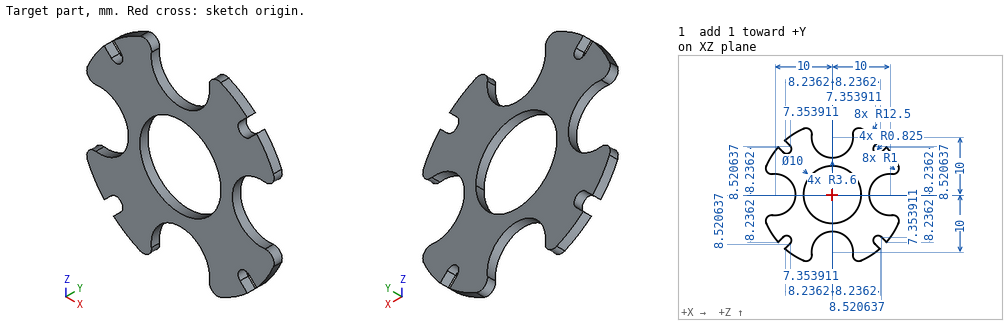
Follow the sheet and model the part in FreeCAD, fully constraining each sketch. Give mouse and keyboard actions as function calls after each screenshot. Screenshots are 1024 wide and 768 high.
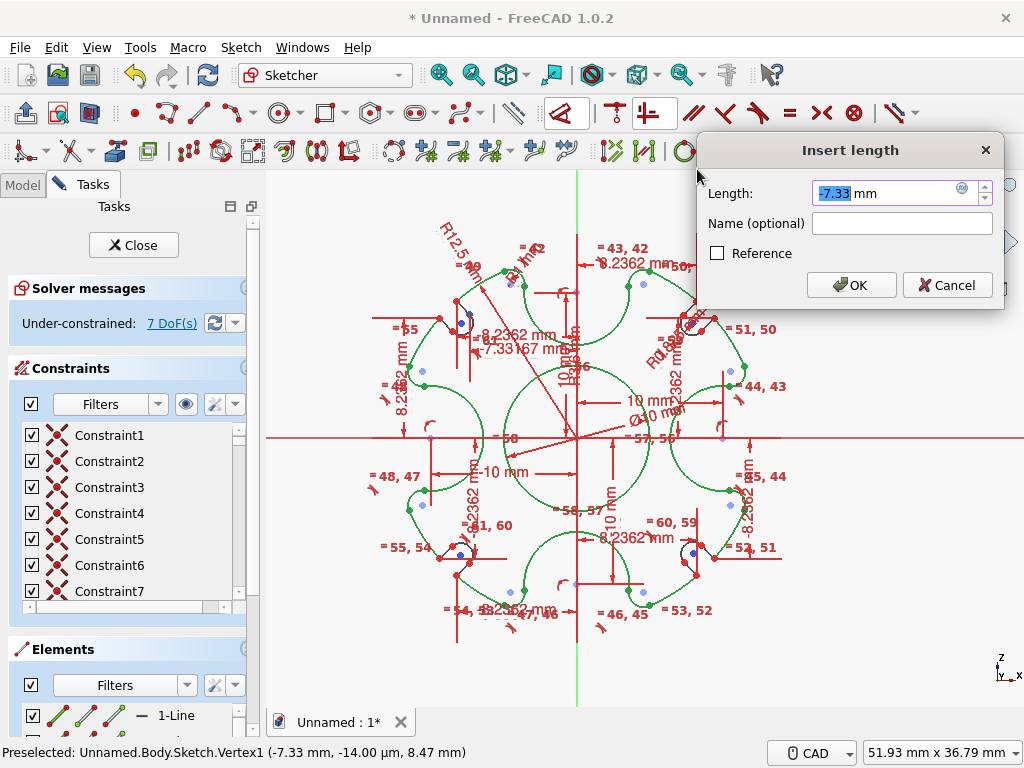
text(-7.353911)
key(Return)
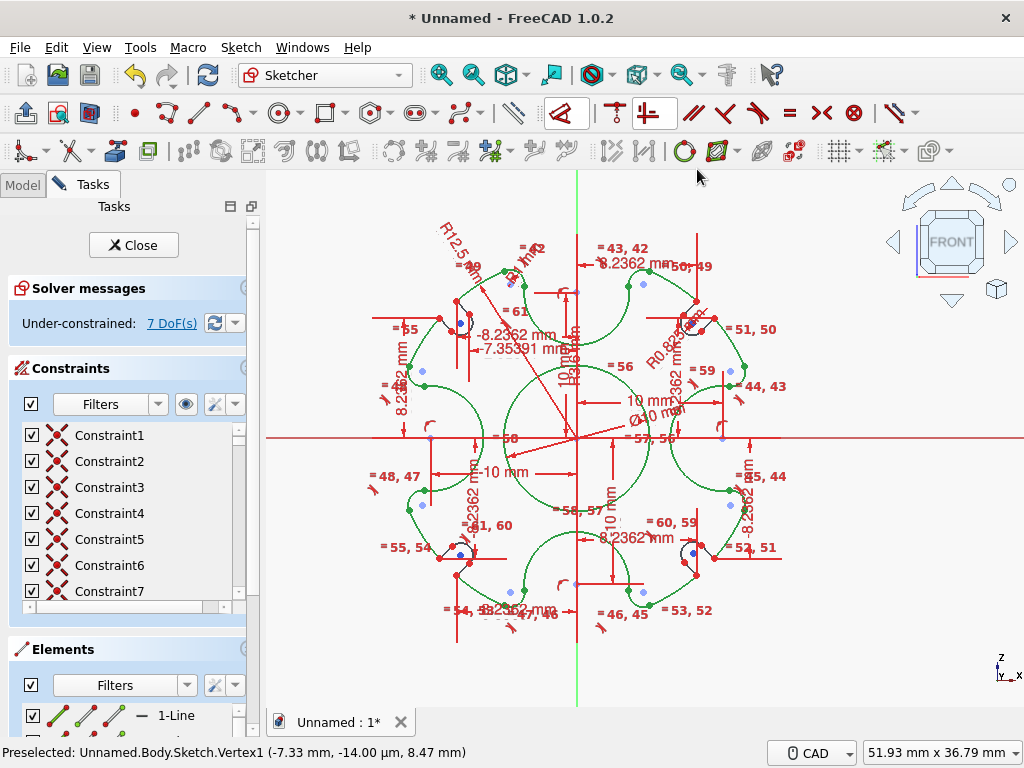
click(469, 315)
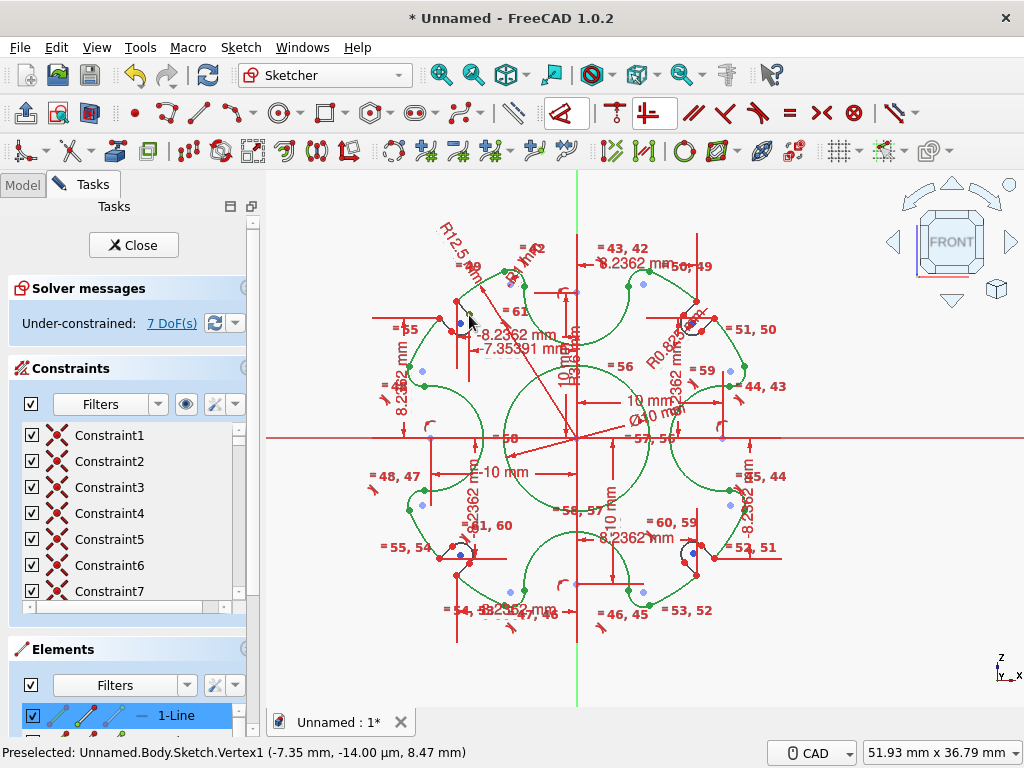
click(584, 114)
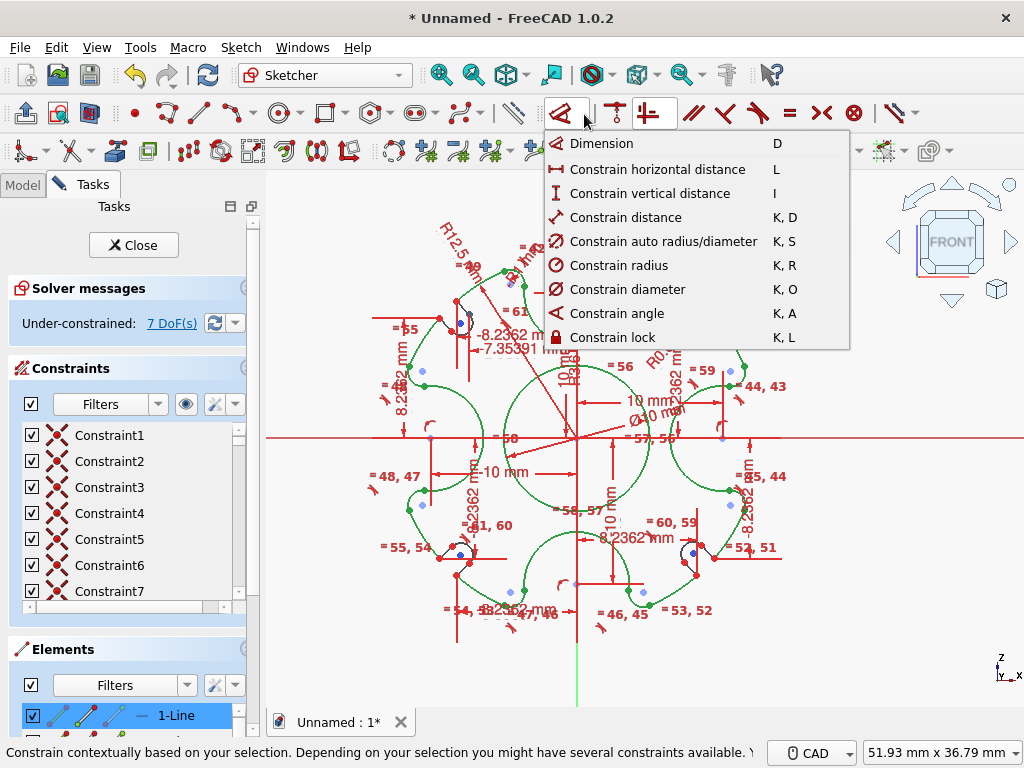
click(697, 193)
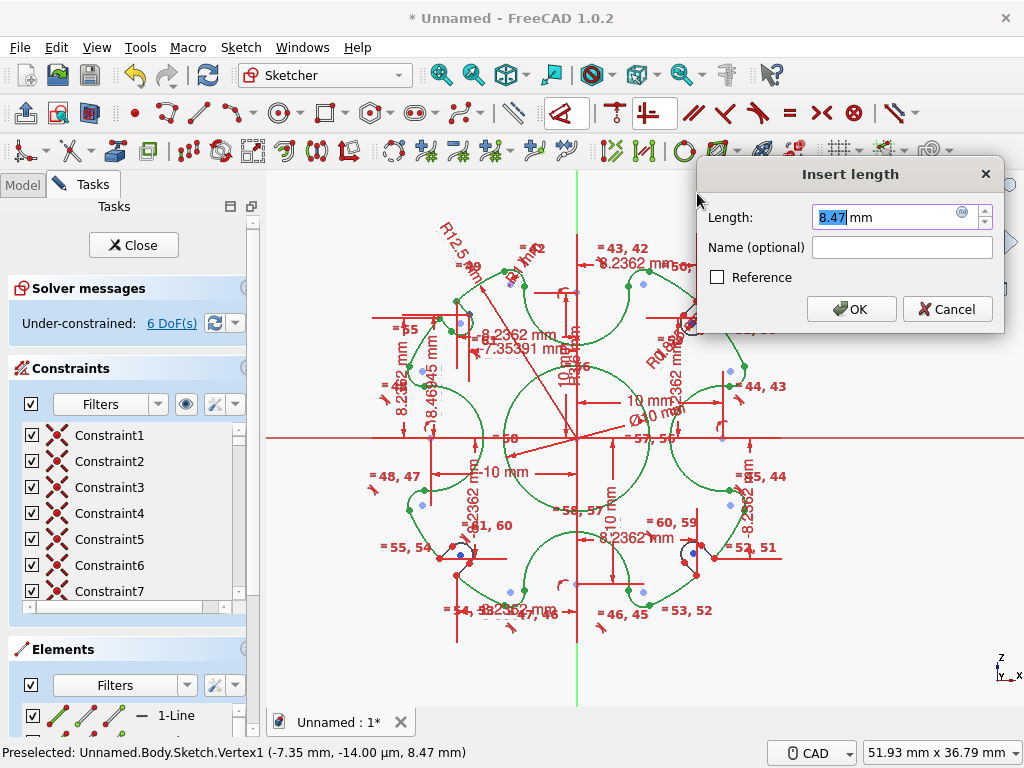
text(8.520637)
key(Return)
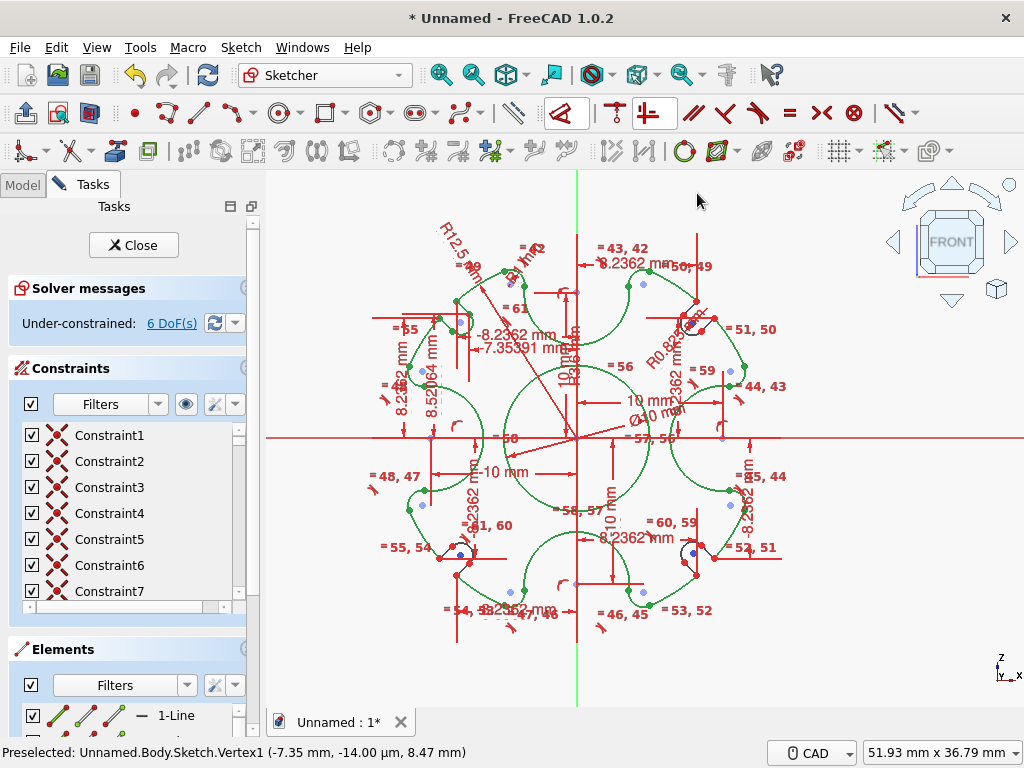
click(684, 315)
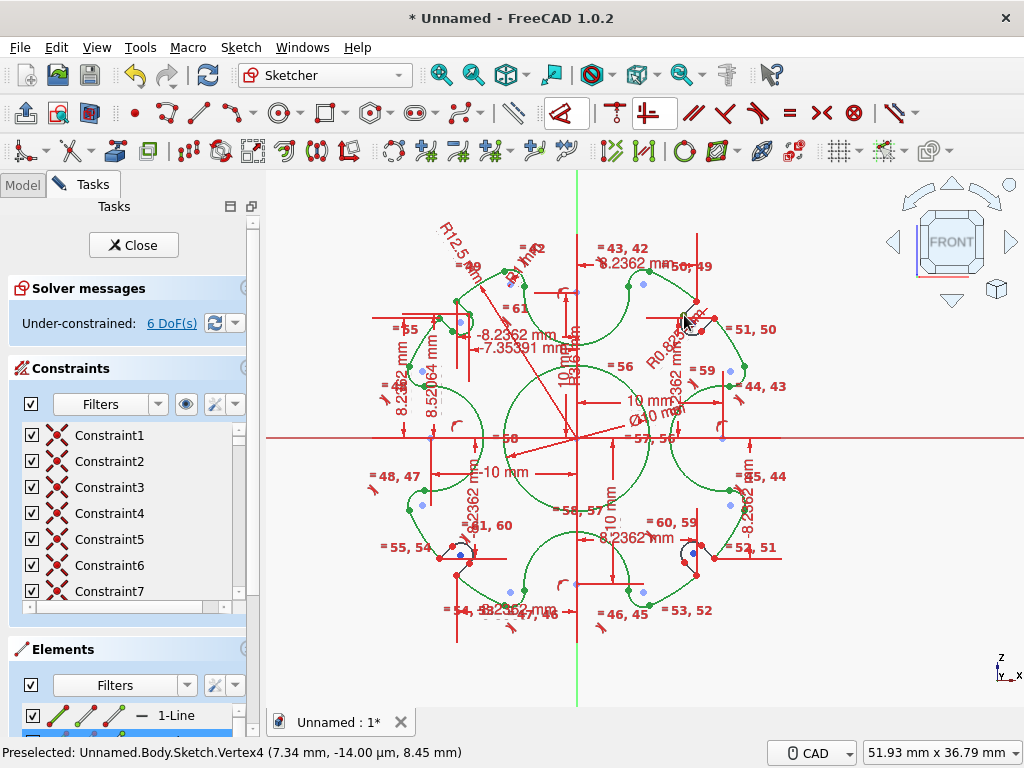
click(584, 114)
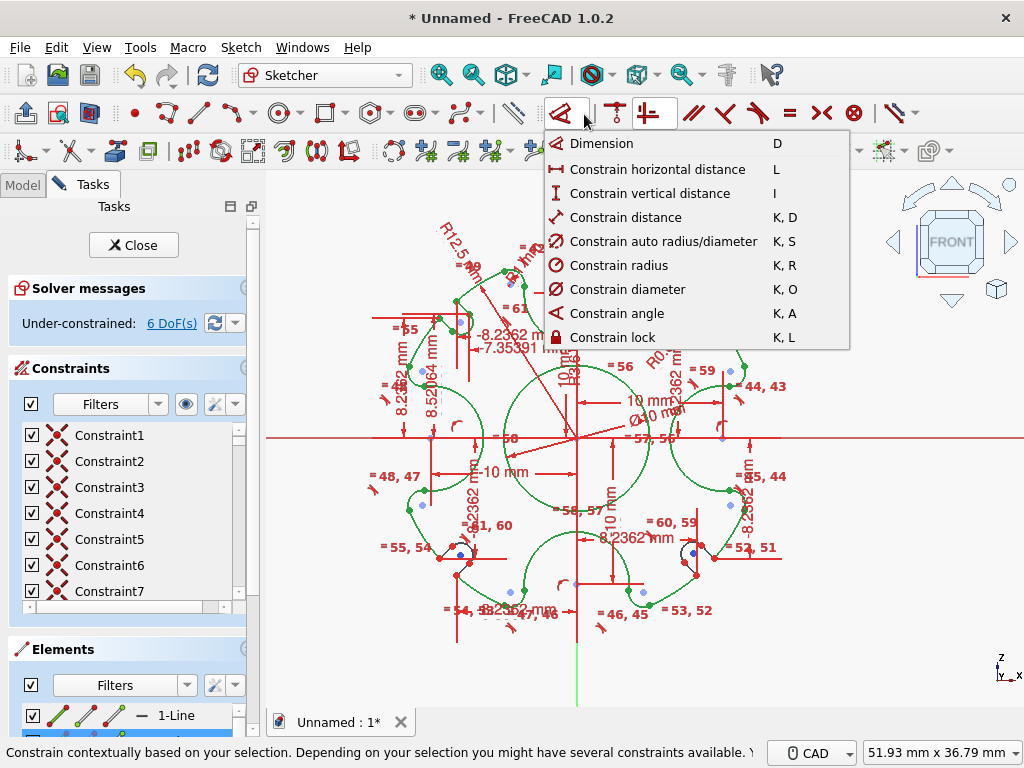
click(697, 169)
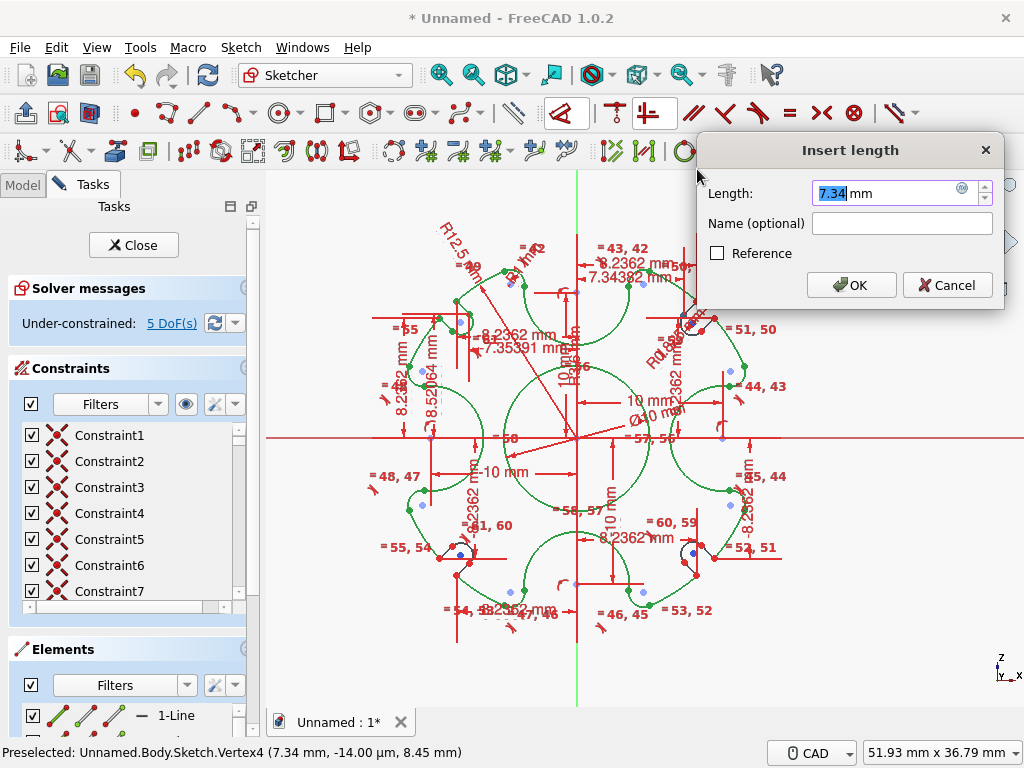
text(7.353911)
key(Return)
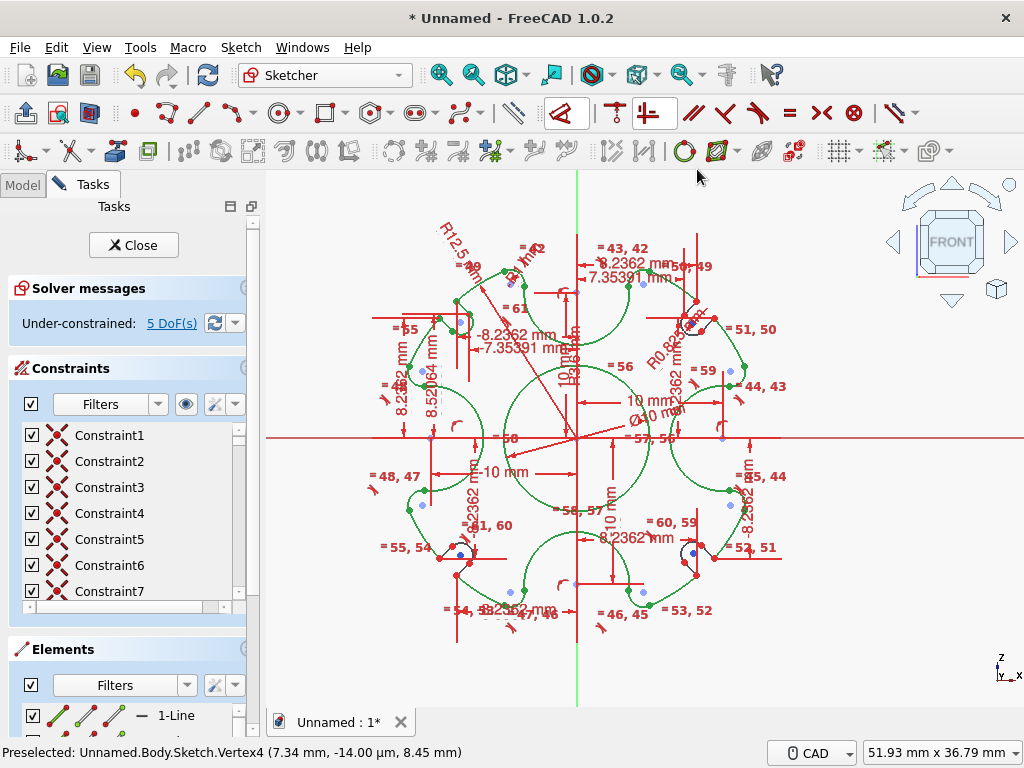
click(684, 315)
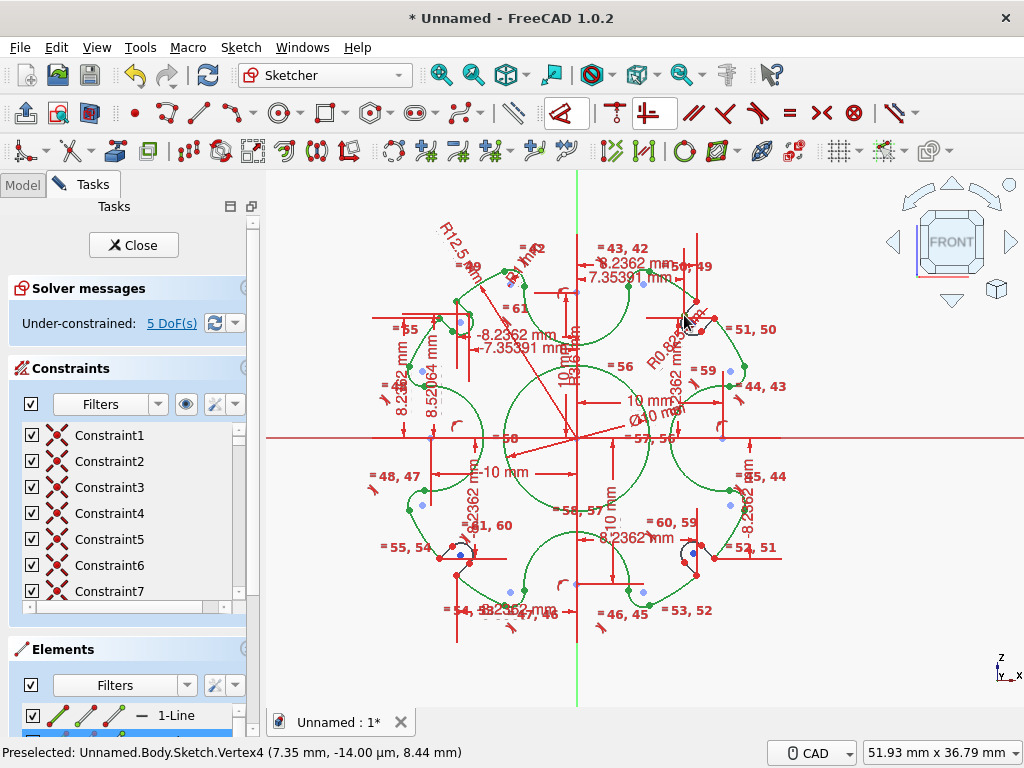
key(i)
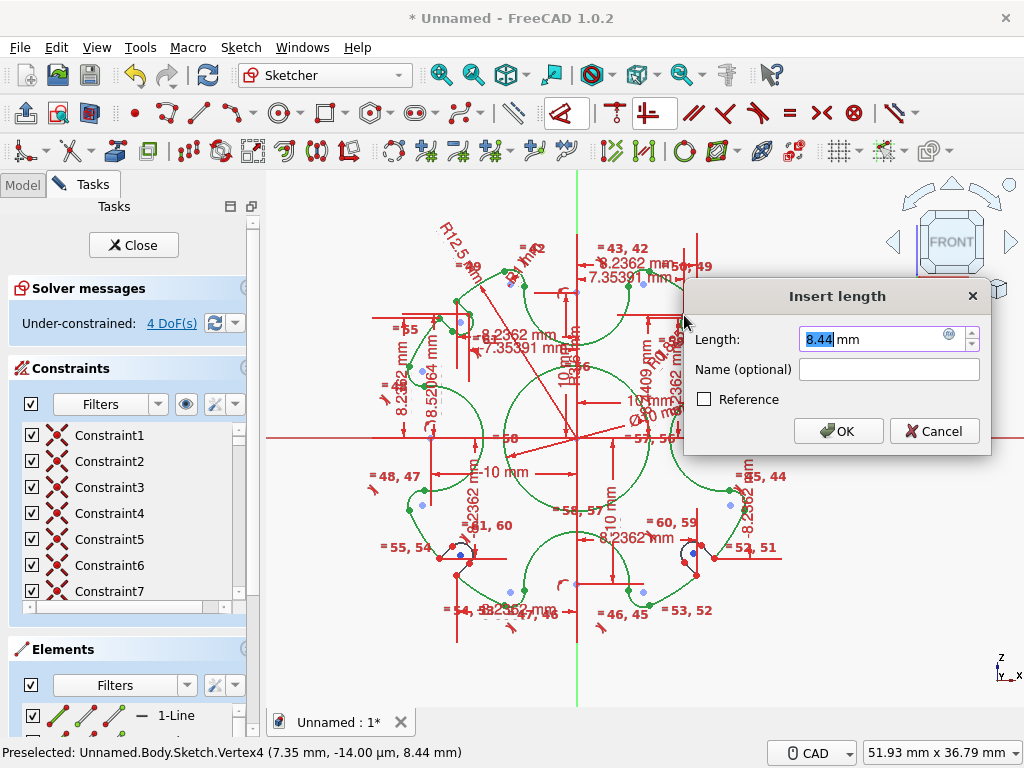
text(8.520637)
key(Return)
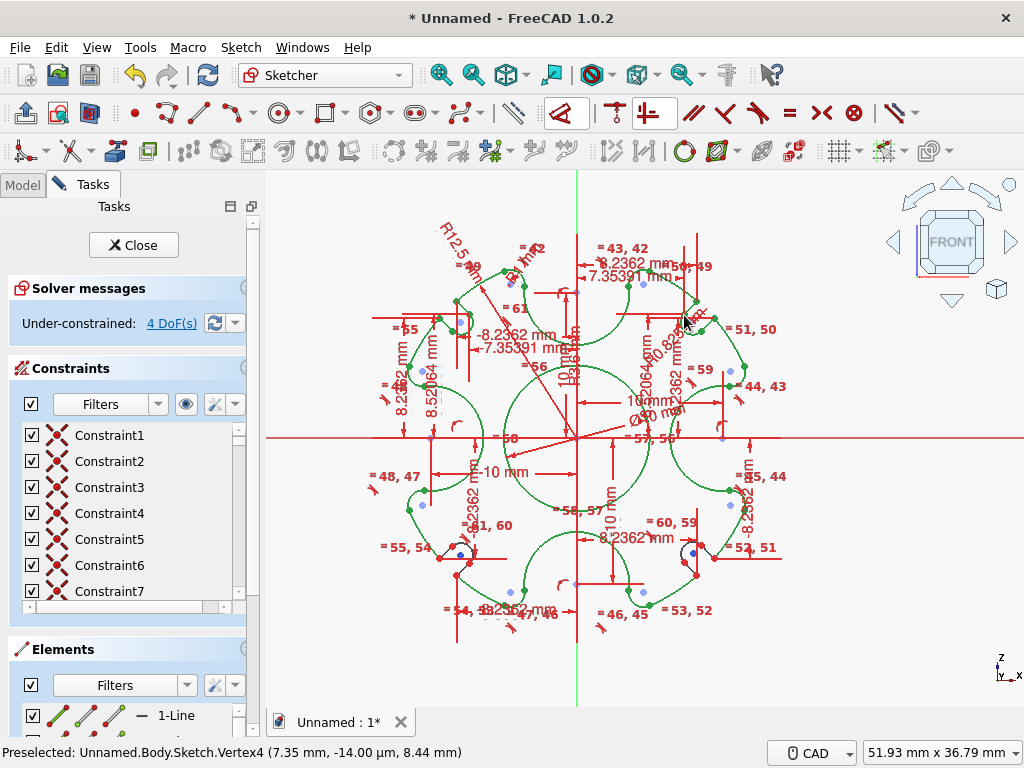
click(702, 546)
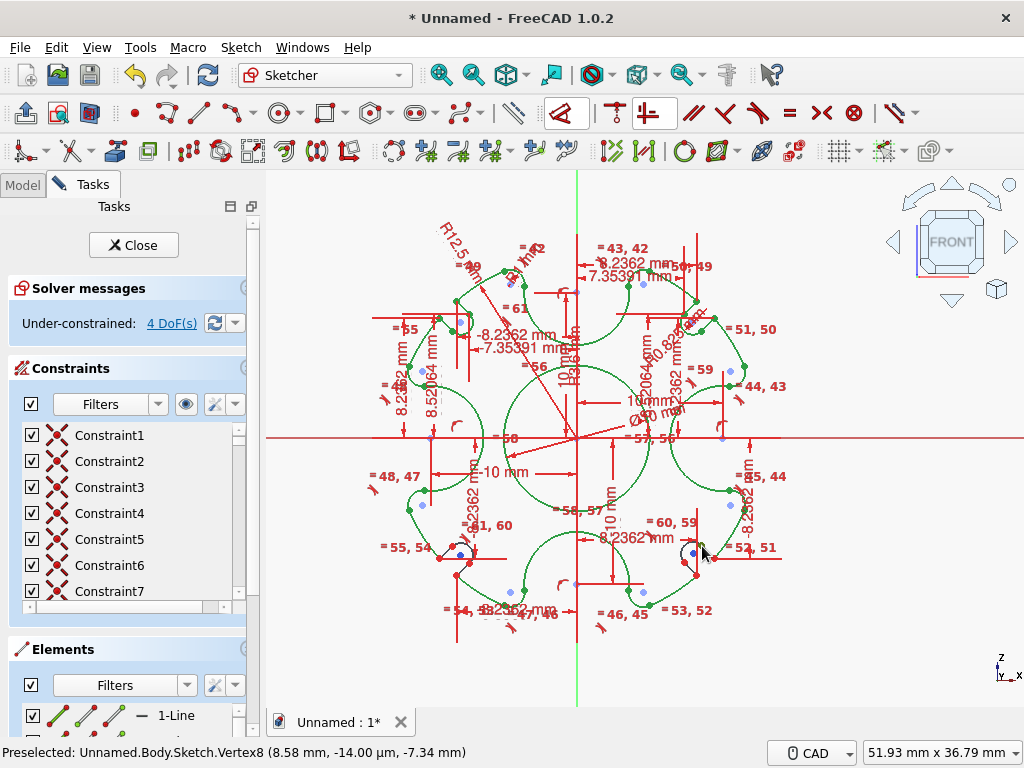
key(l)